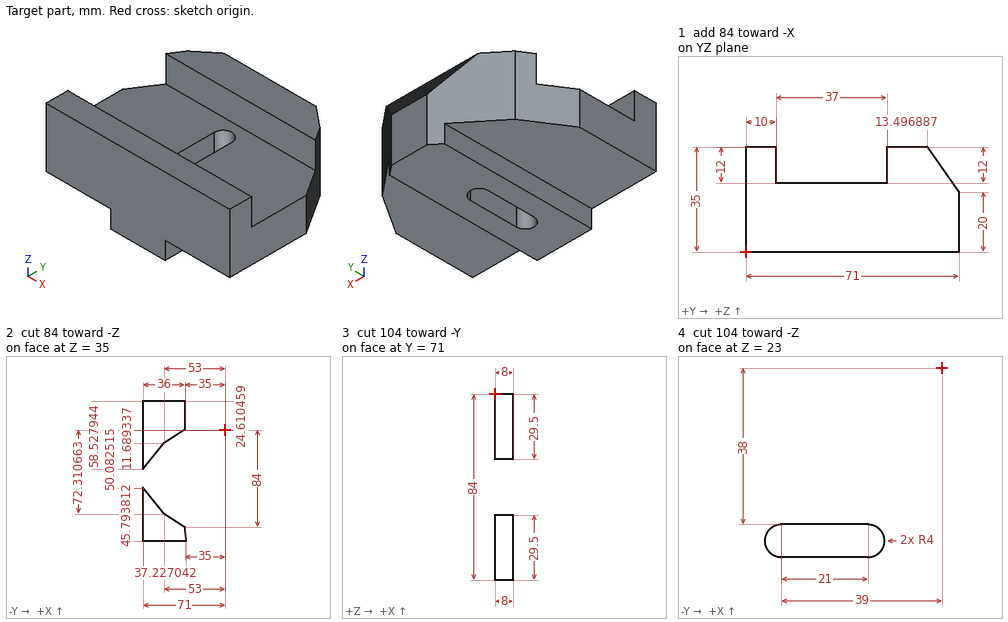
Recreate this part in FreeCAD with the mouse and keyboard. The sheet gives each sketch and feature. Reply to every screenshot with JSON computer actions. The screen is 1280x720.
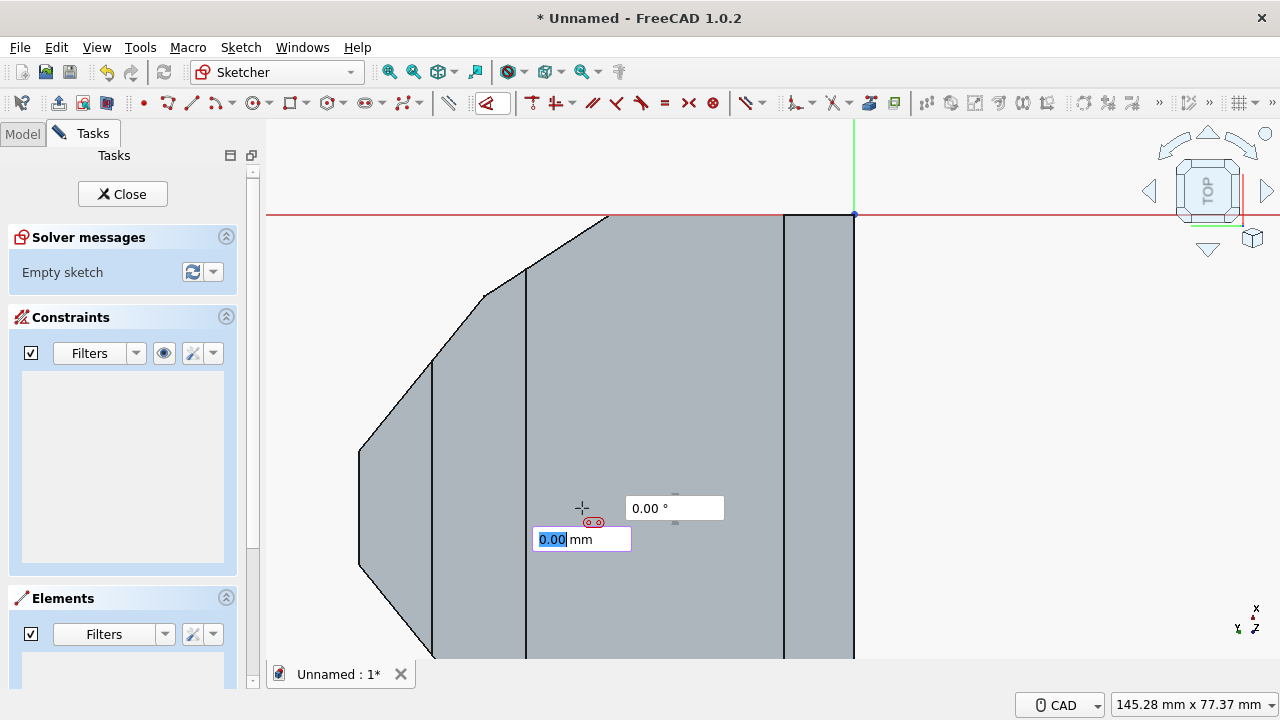
{"action": "left_click", "coordinate": [729, 508]}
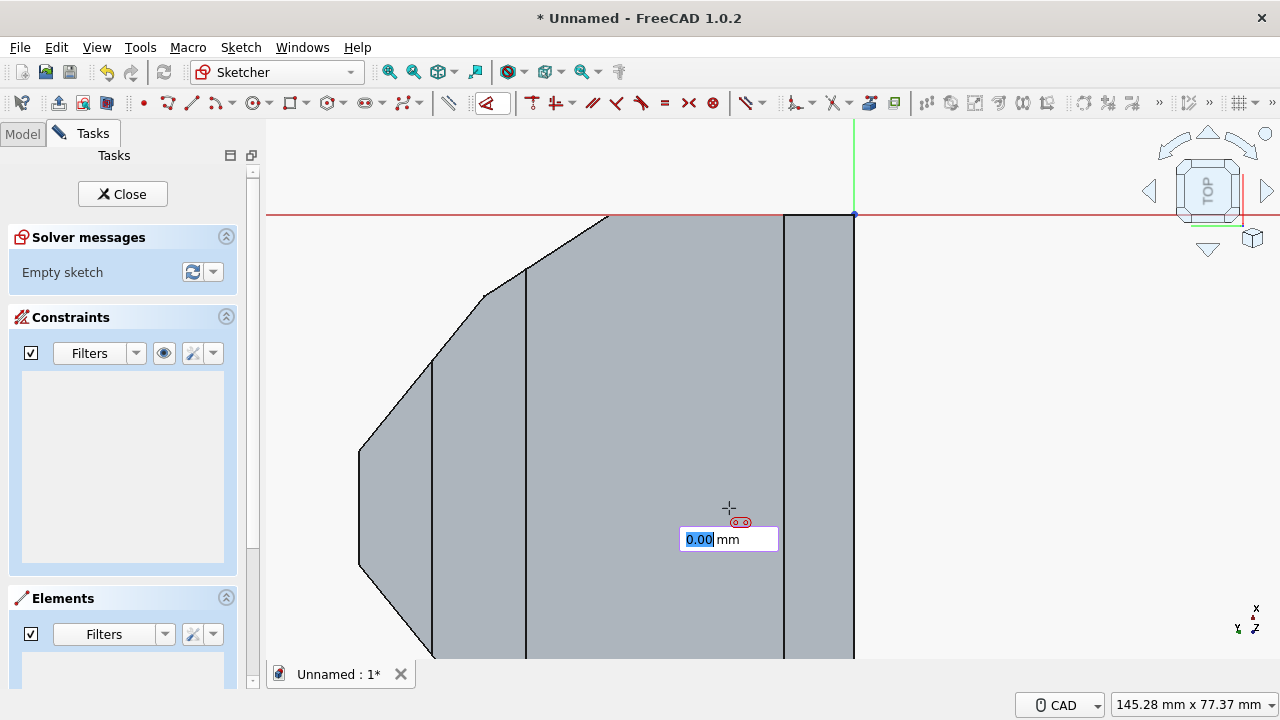
{"action": "left_click", "coordinate": [655, 536]}
{"action": "key", "text": "Escape"}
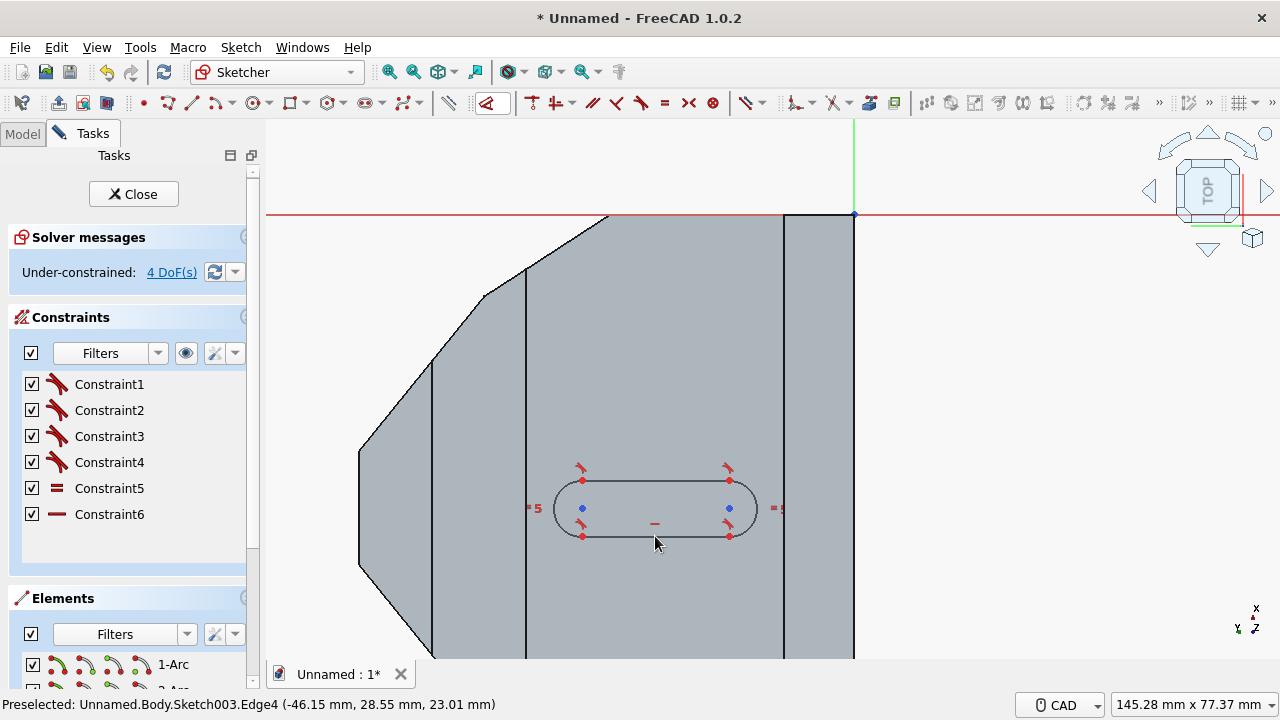
{"action": "scroll", "coordinate": [559, 493], "scroll_direction": "up", "scroll_amount": 2}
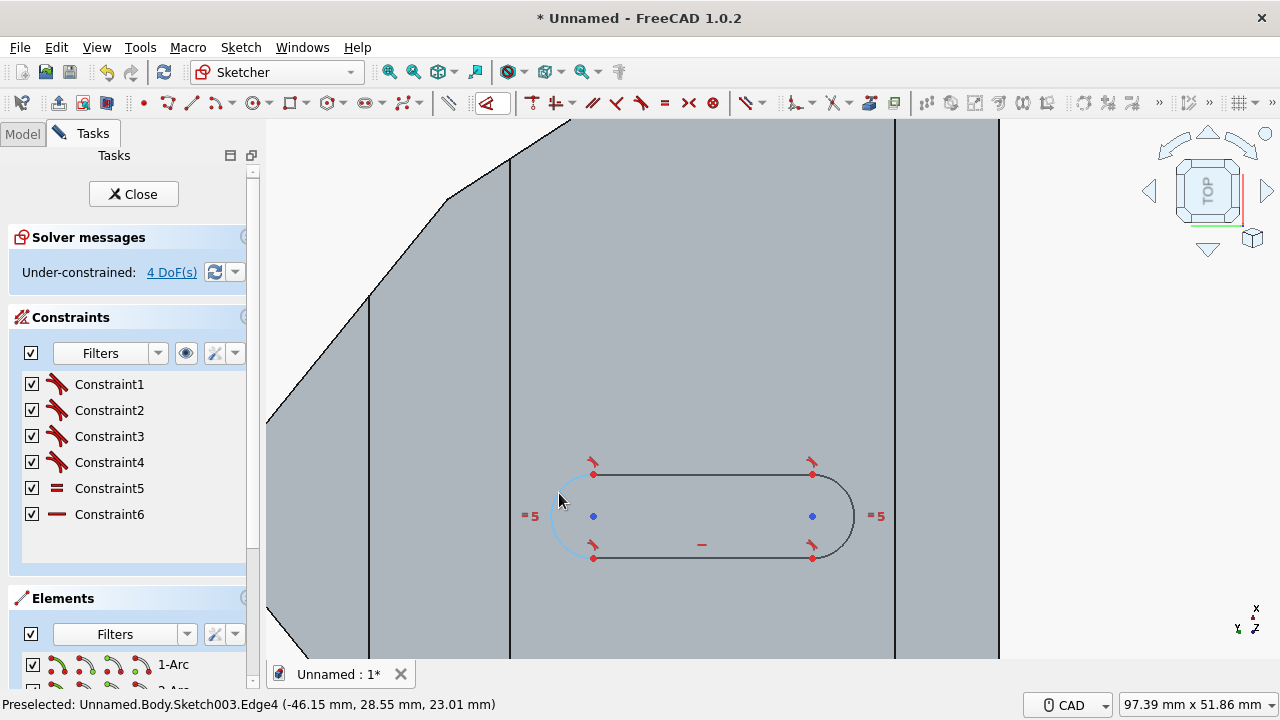
{"action": "left_click", "coordinate": [559, 492]}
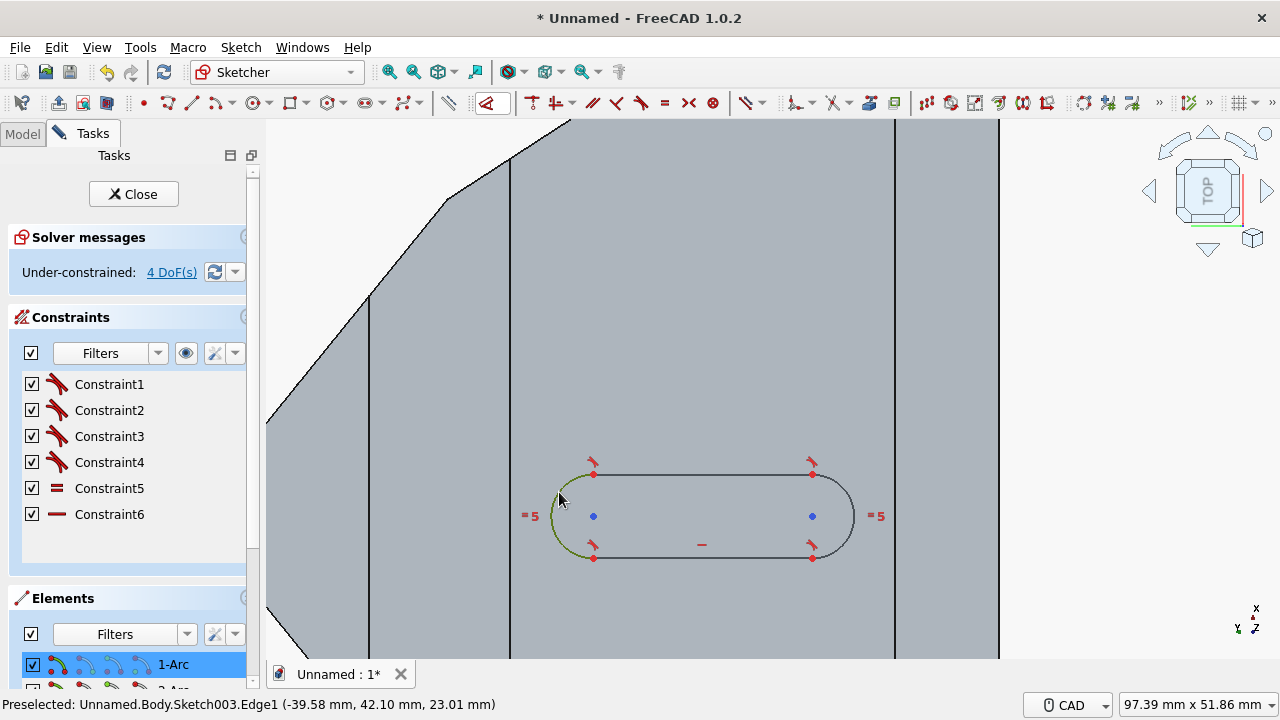
{"action": "left_click", "coordinate": [504, 104]}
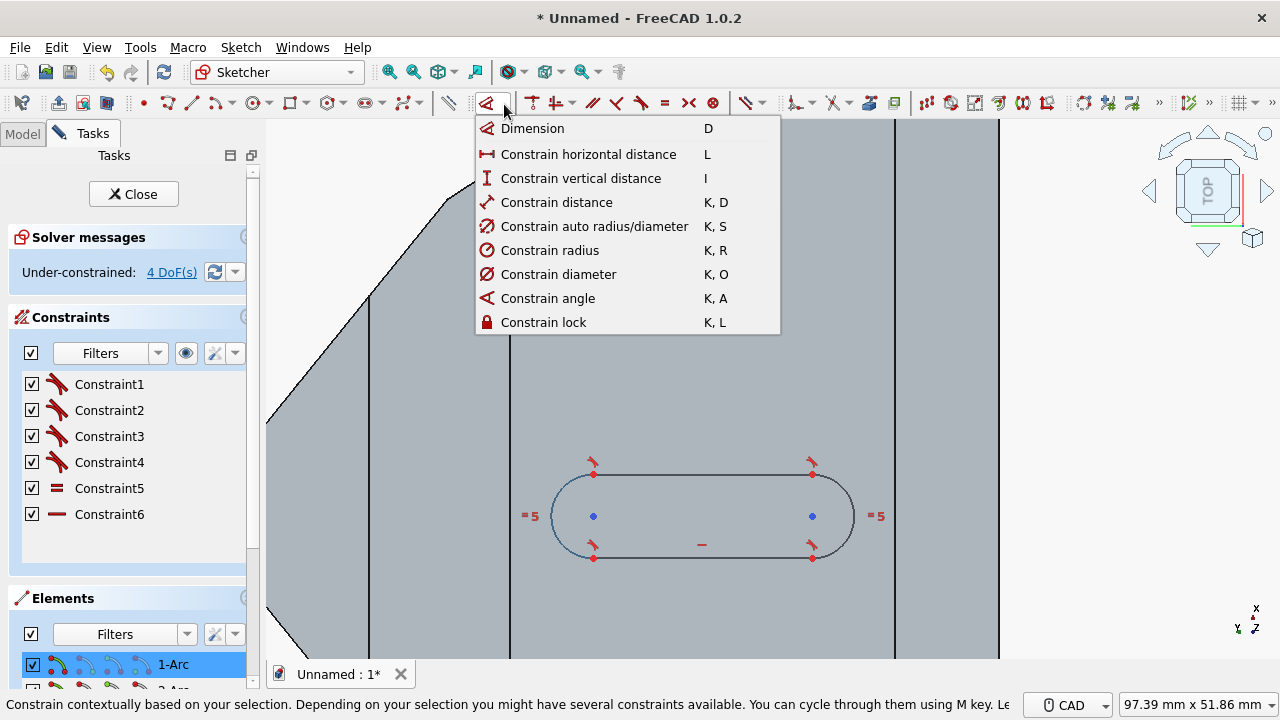
{"action": "left_click", "coordinate": [628, 250]}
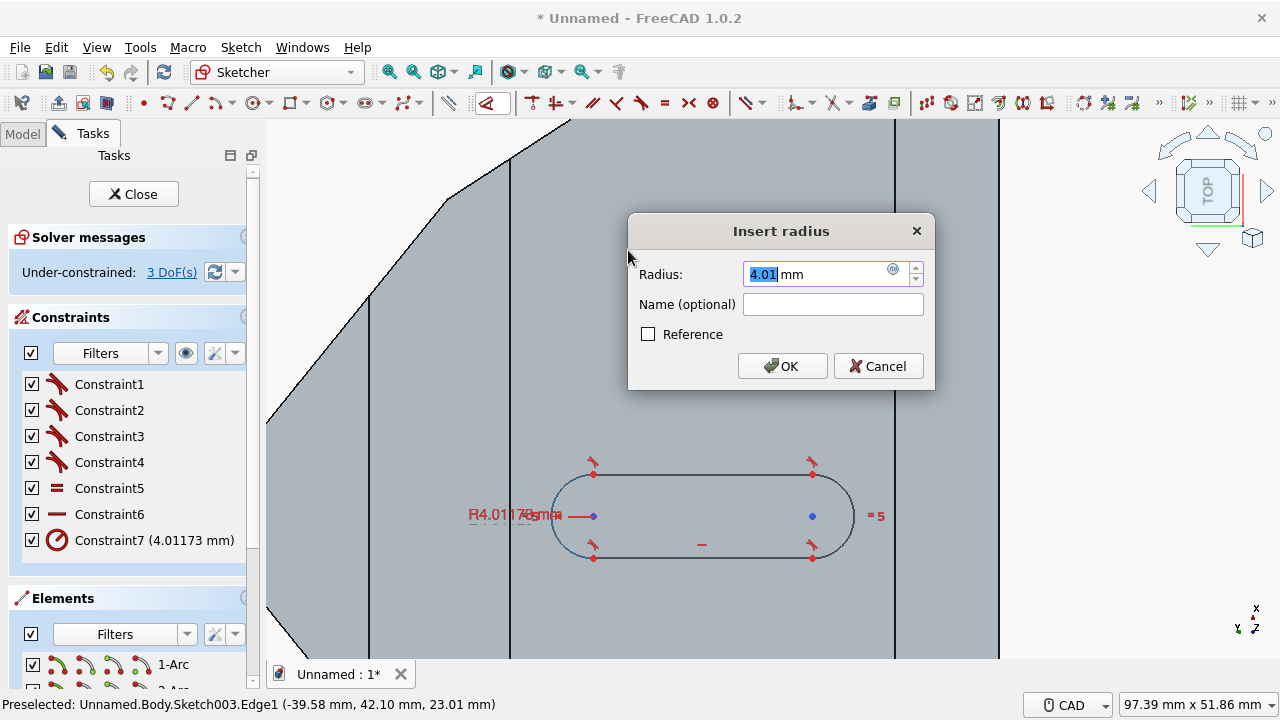
{"action": "type", "text": "4"}
{"action": "key", "text": "Return"}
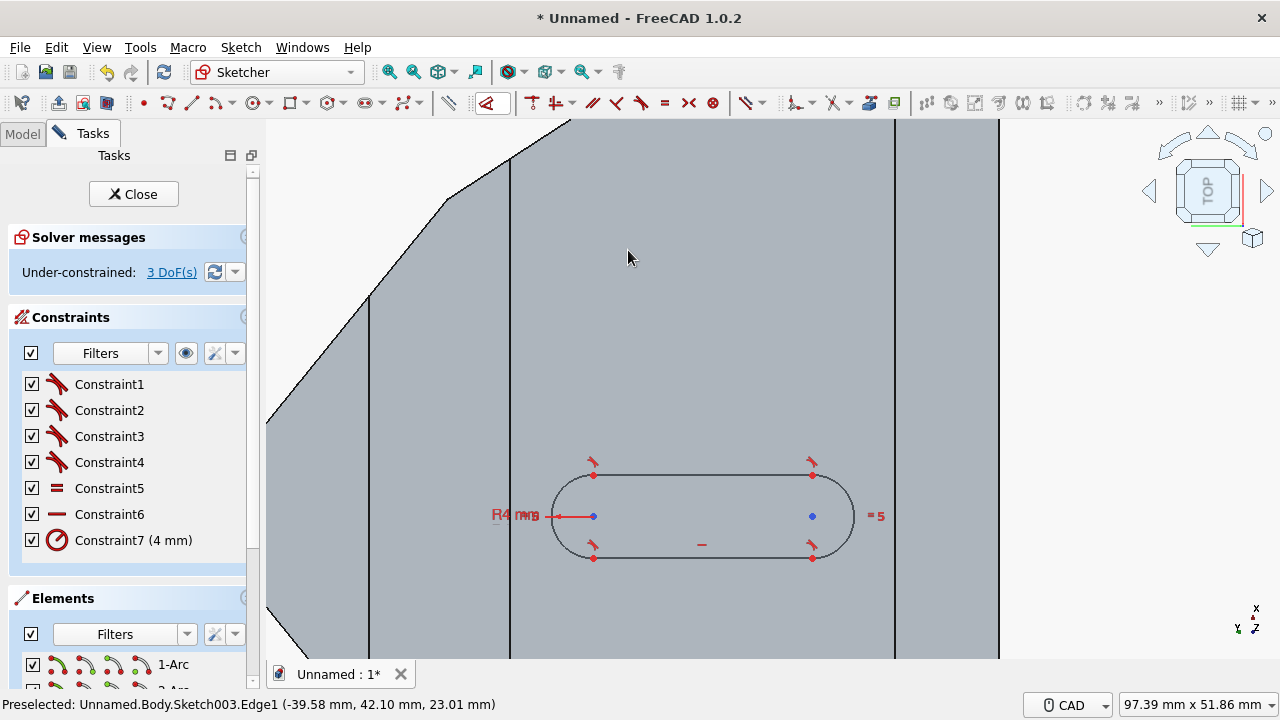
{"action": "left_click", "coordinate": [659, 475]}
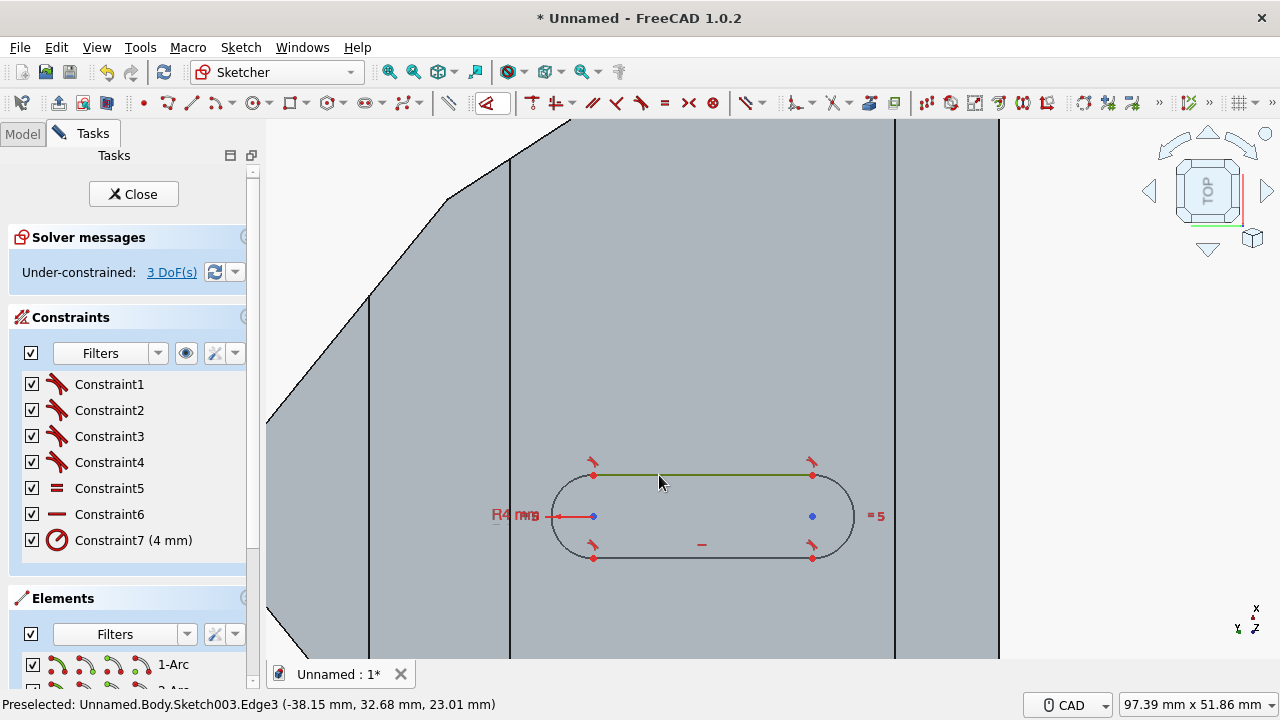
{"action": "left_click", "coordinate": [504, 104]}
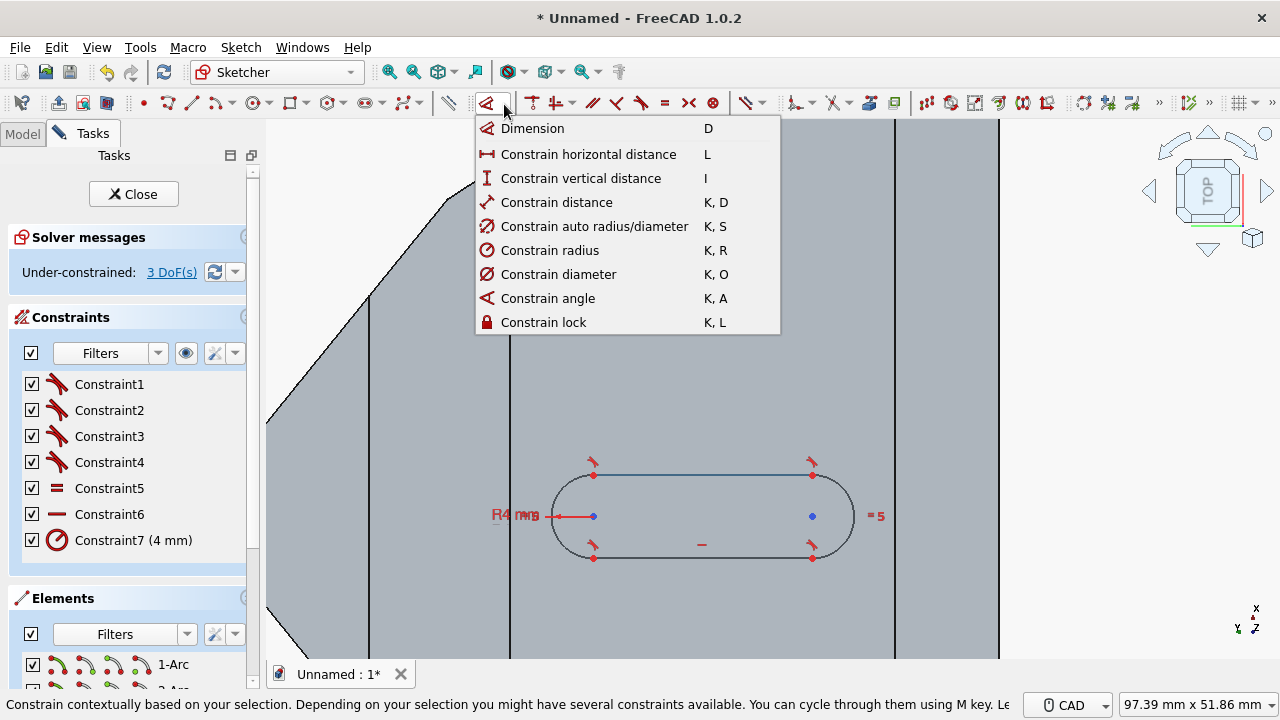
{"action": "left_click", "coordinate": [628, 154]}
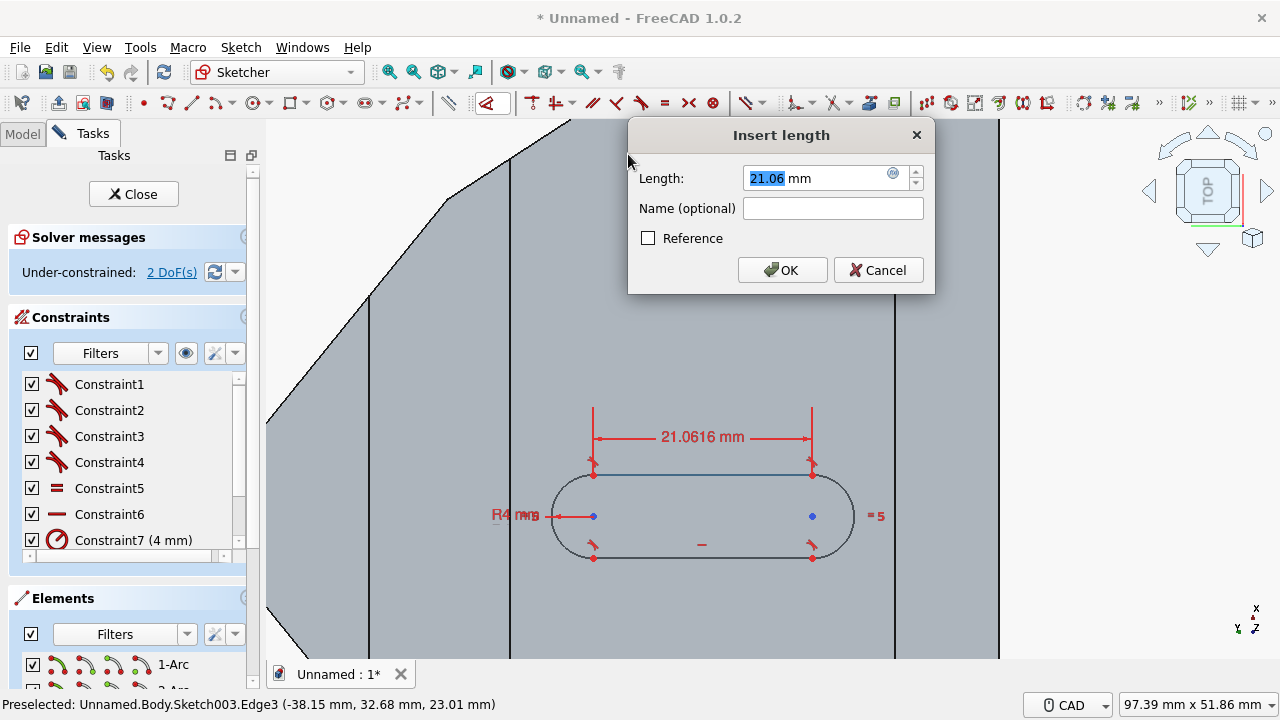
{"action": "type", "text": "21"}
{"action": "key", "text": "Return"}